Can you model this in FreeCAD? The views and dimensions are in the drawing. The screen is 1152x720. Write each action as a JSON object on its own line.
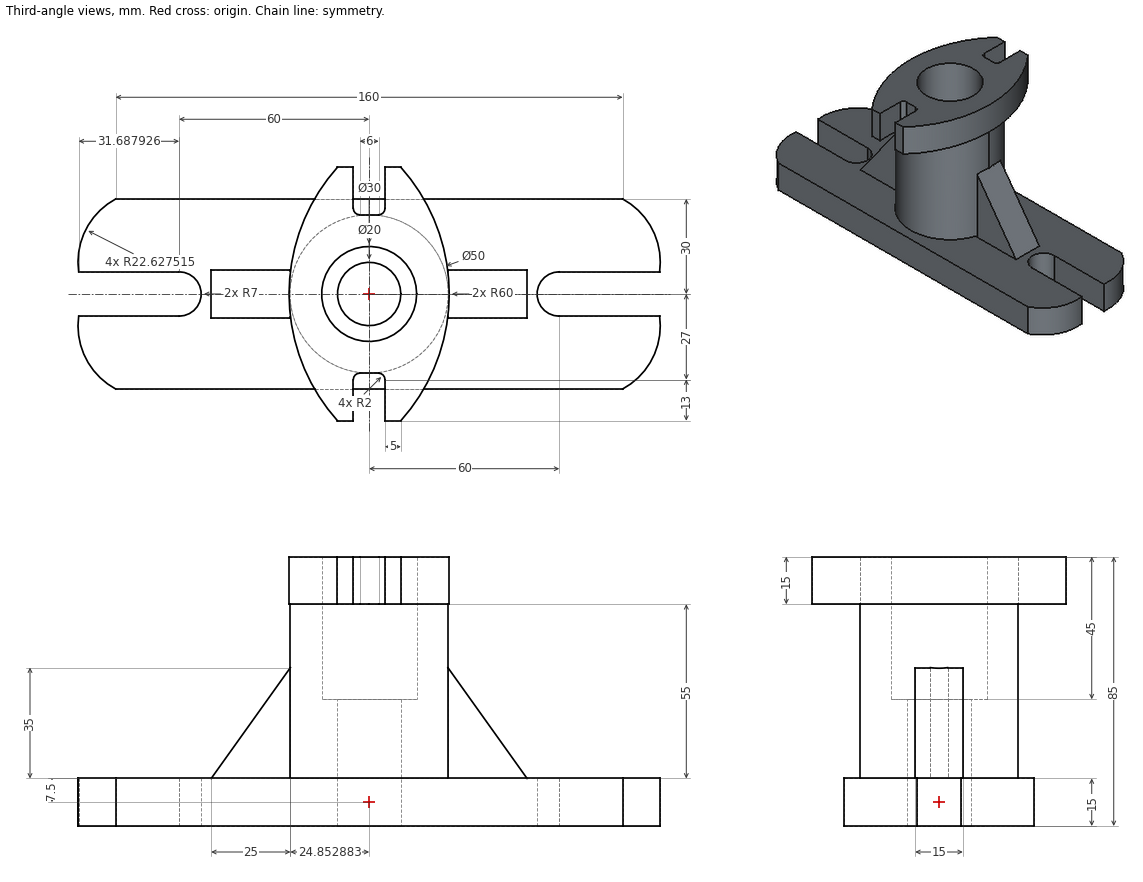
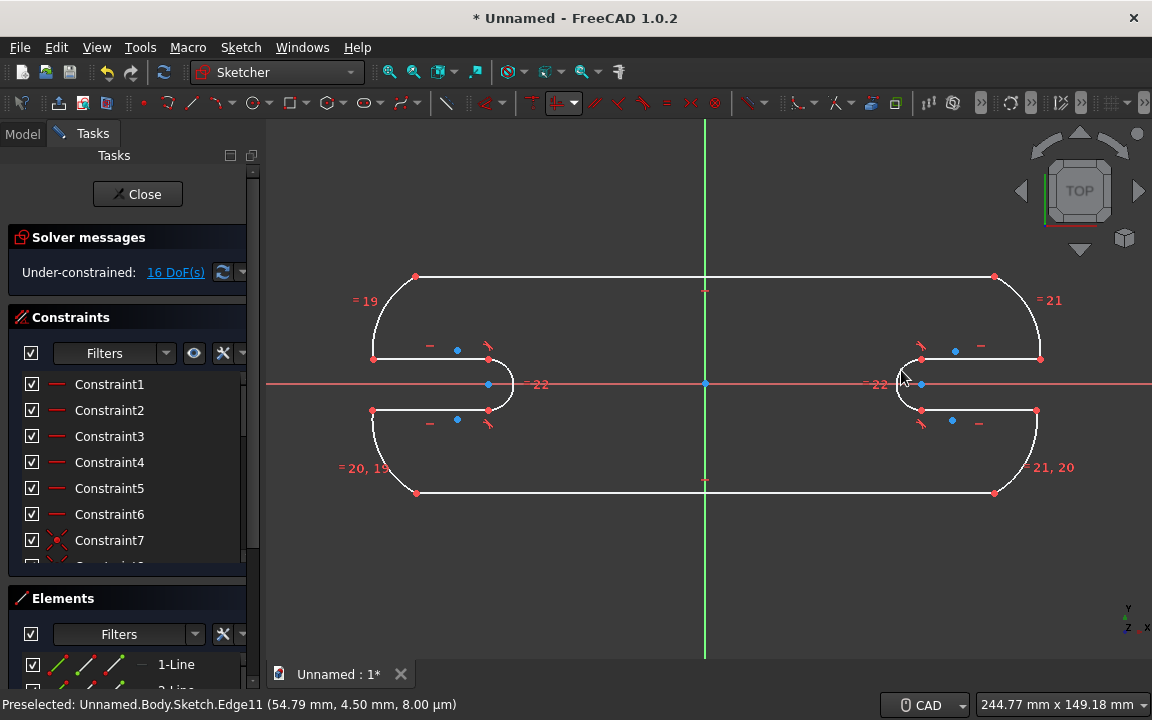
{"action": "left_click", "coordinate": [488, 385]}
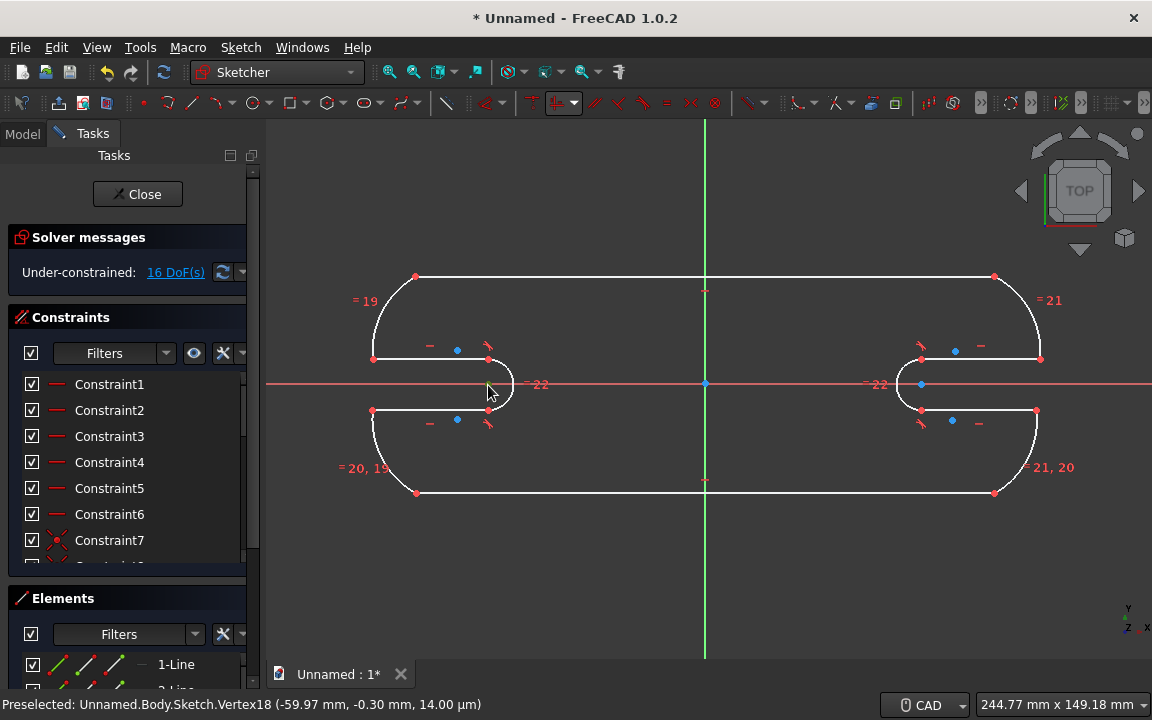
{"action": "left_click", "coordinate": [344, 384]}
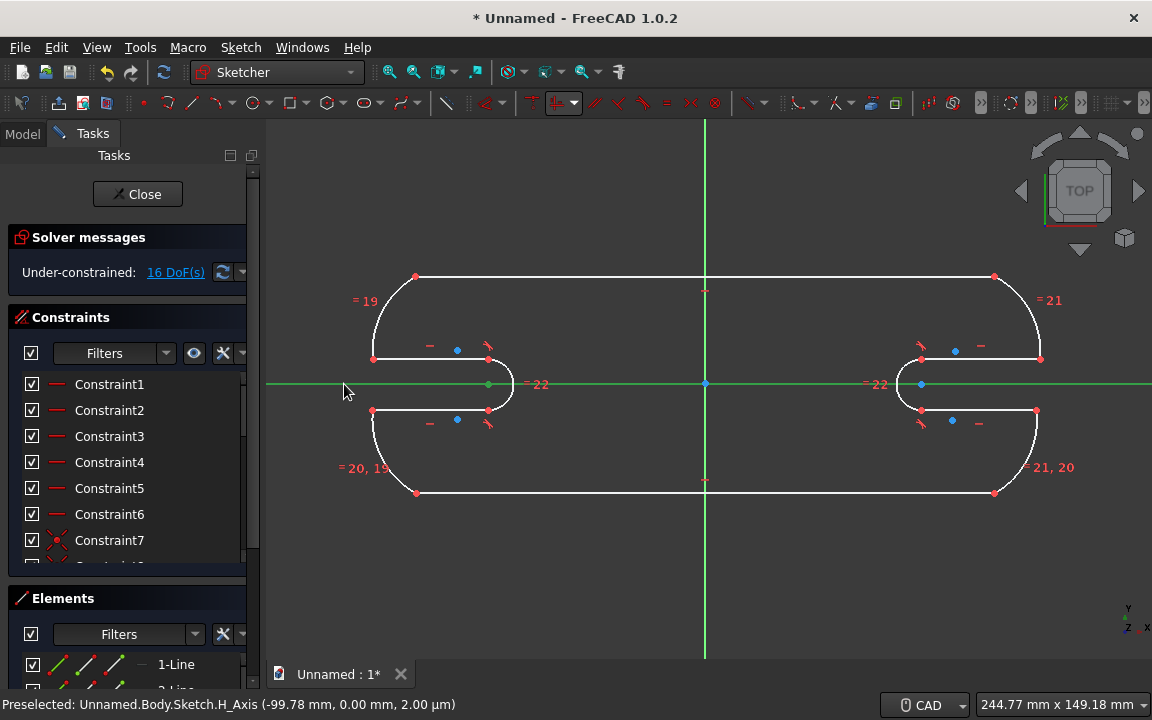
{"action": "key", "text": "c"}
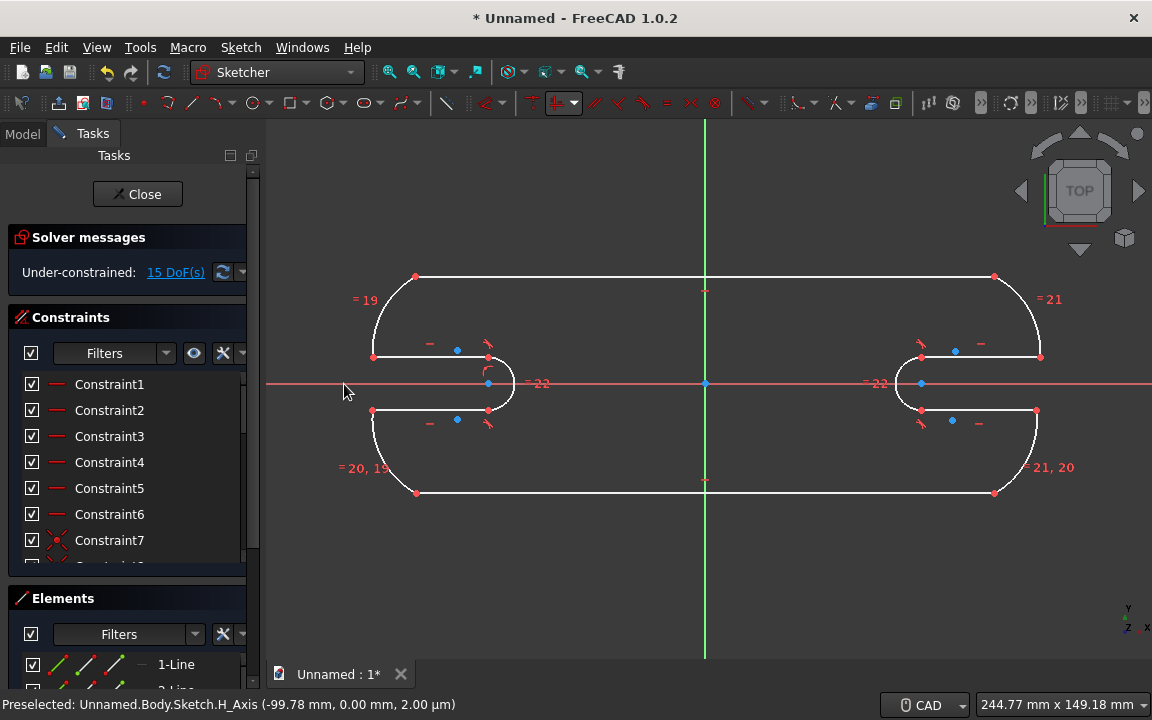
{"action": "left_click", "coordinate": [922, 384]}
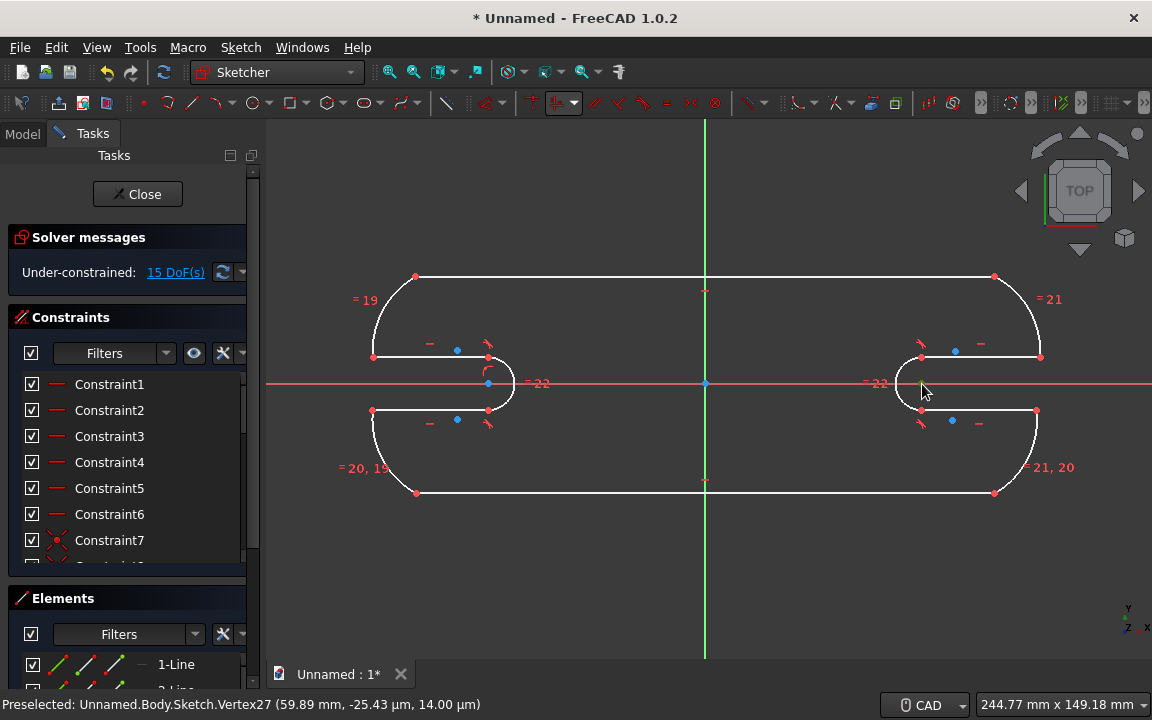
{"action": "left_click", "coordinate": [344, 384]}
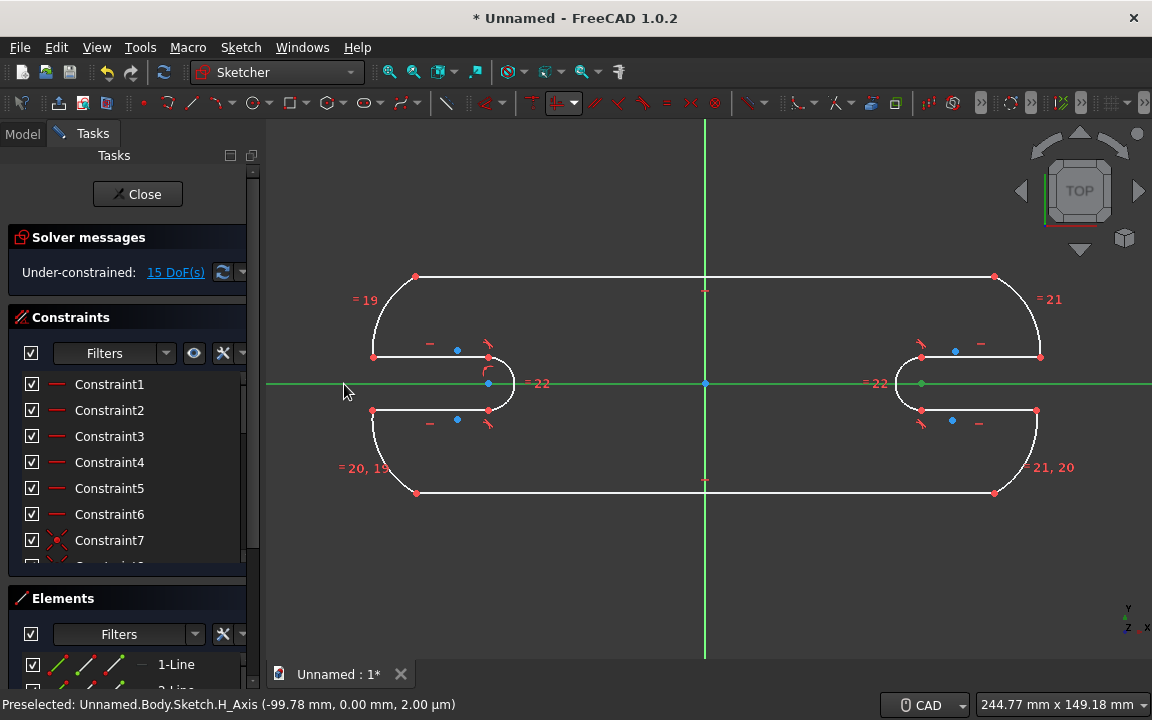
{"action": "left_click", "coordinate": [532, 104]}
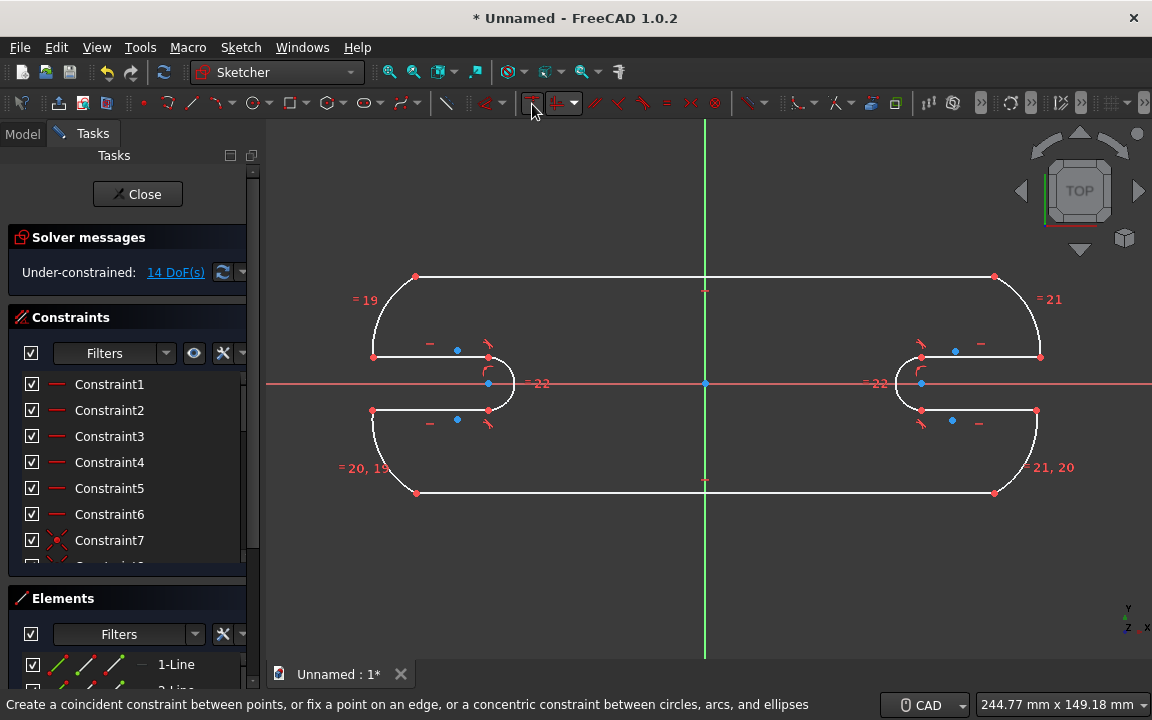
{"action": "left_click", "coordinate": [458, 351]}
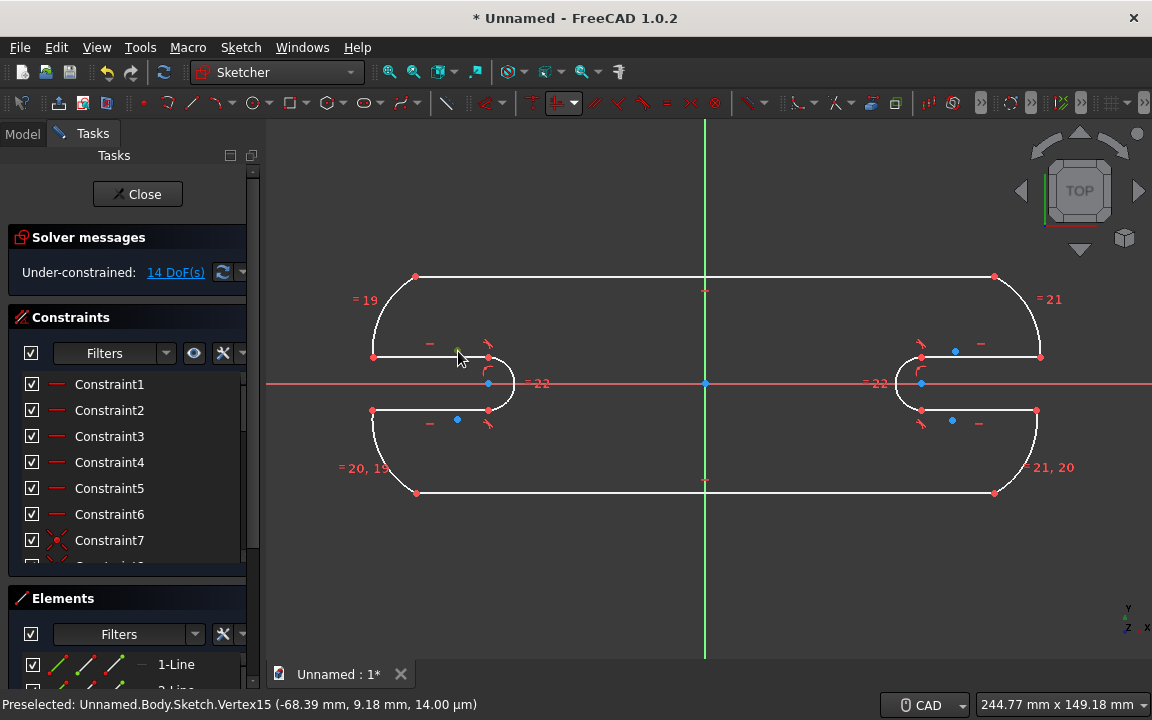
{"action": "left_click", "coordinate": [457, 419]}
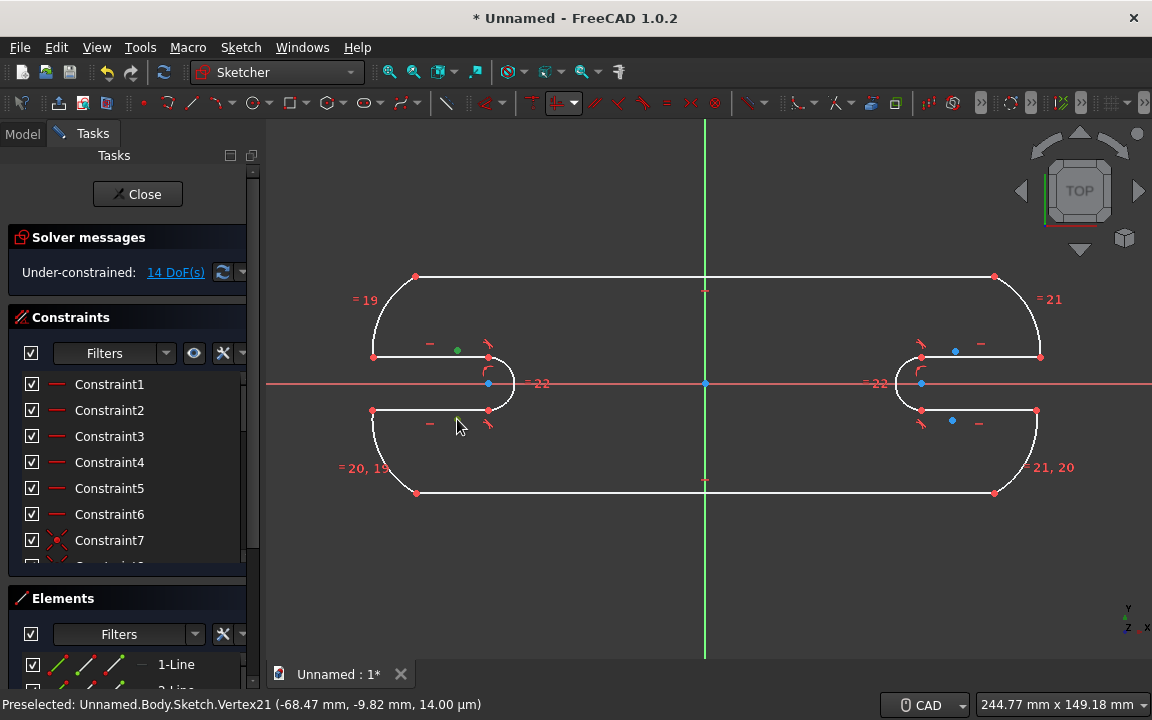
{"action": "left_click", "coordinate": [344, 384]}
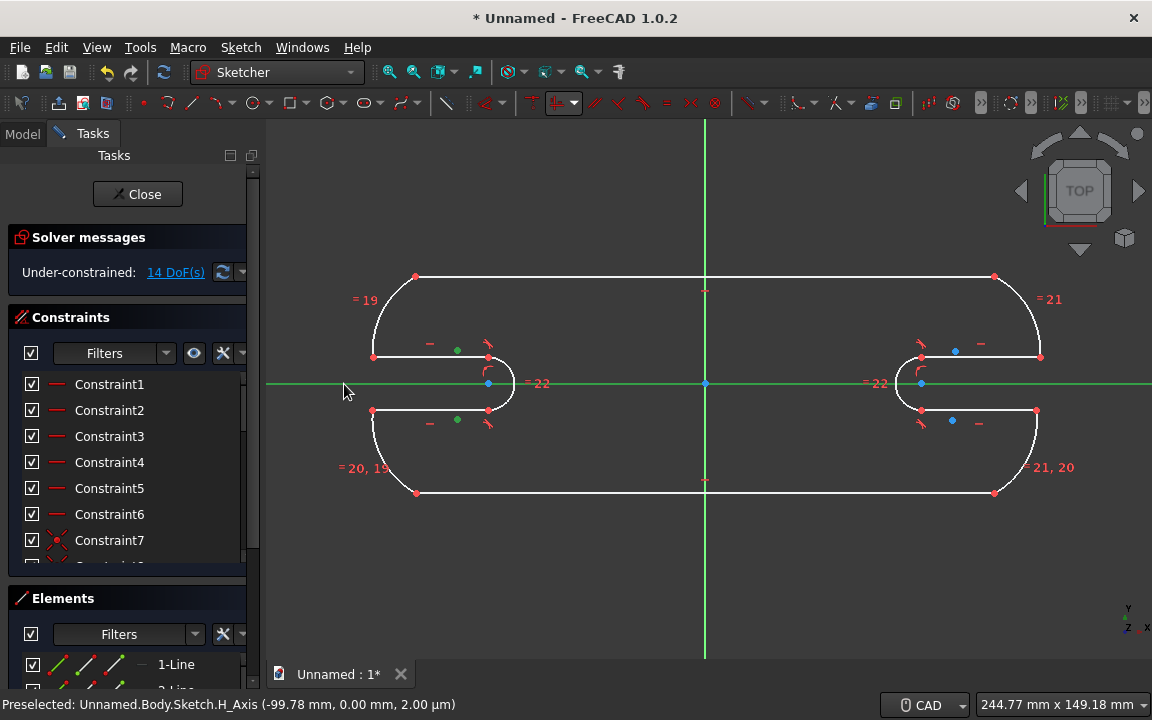
{"action": "key", "text": "s"}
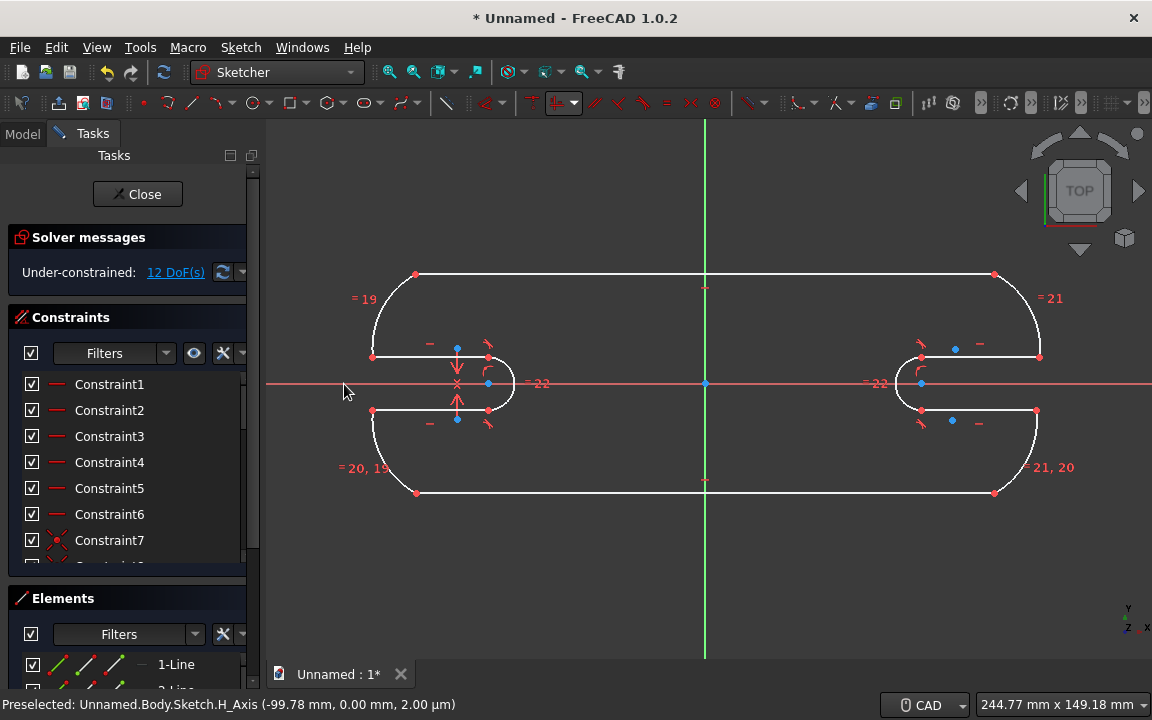
{"action": "left_click", "coordinate": [457, 419]}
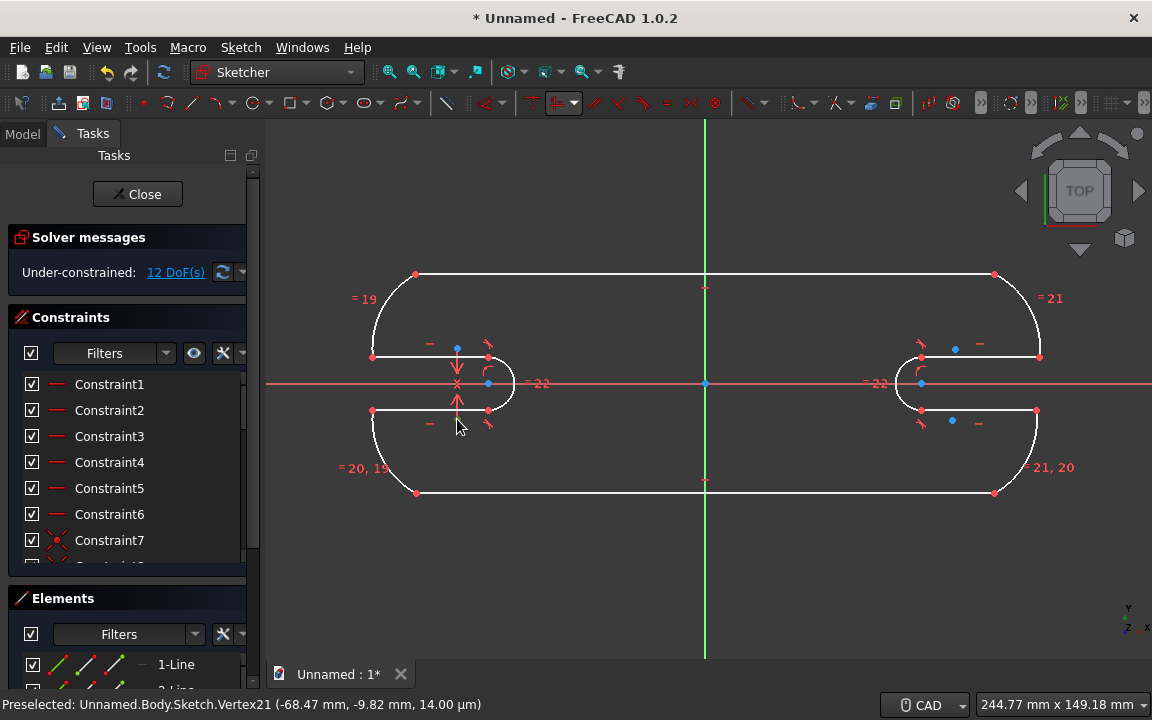
{"action": "left_click", "coordinate": [952, 420]}